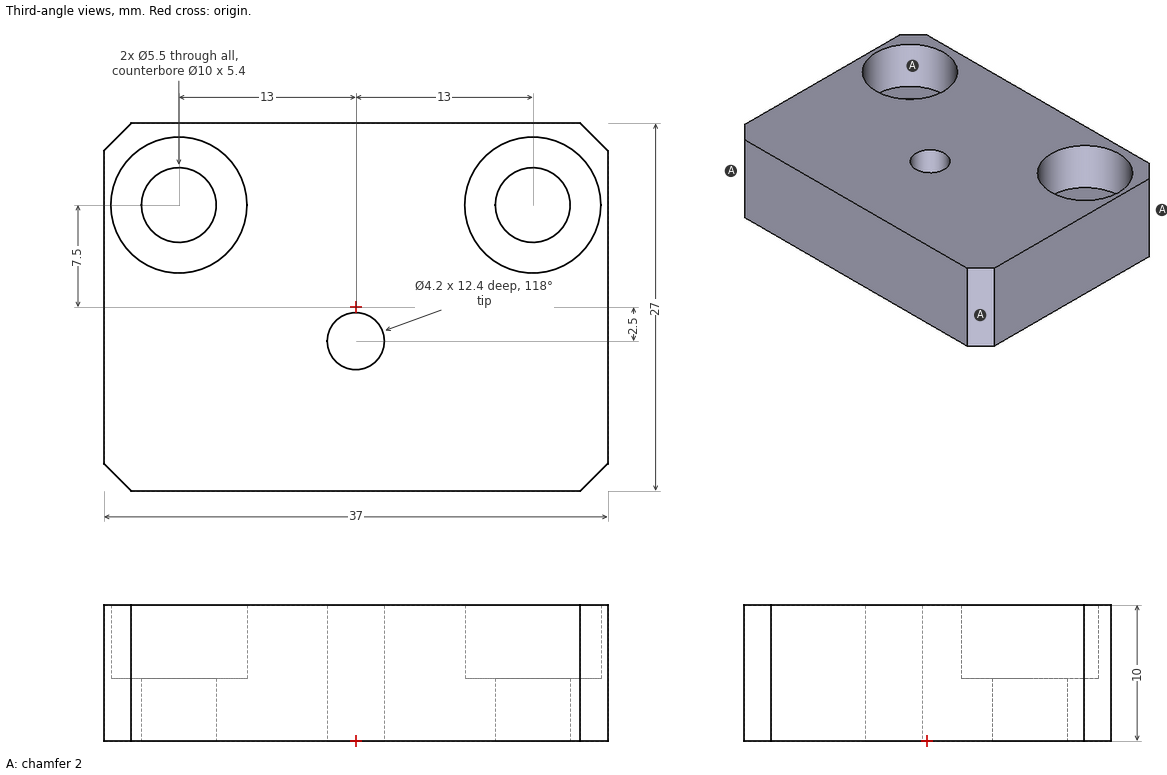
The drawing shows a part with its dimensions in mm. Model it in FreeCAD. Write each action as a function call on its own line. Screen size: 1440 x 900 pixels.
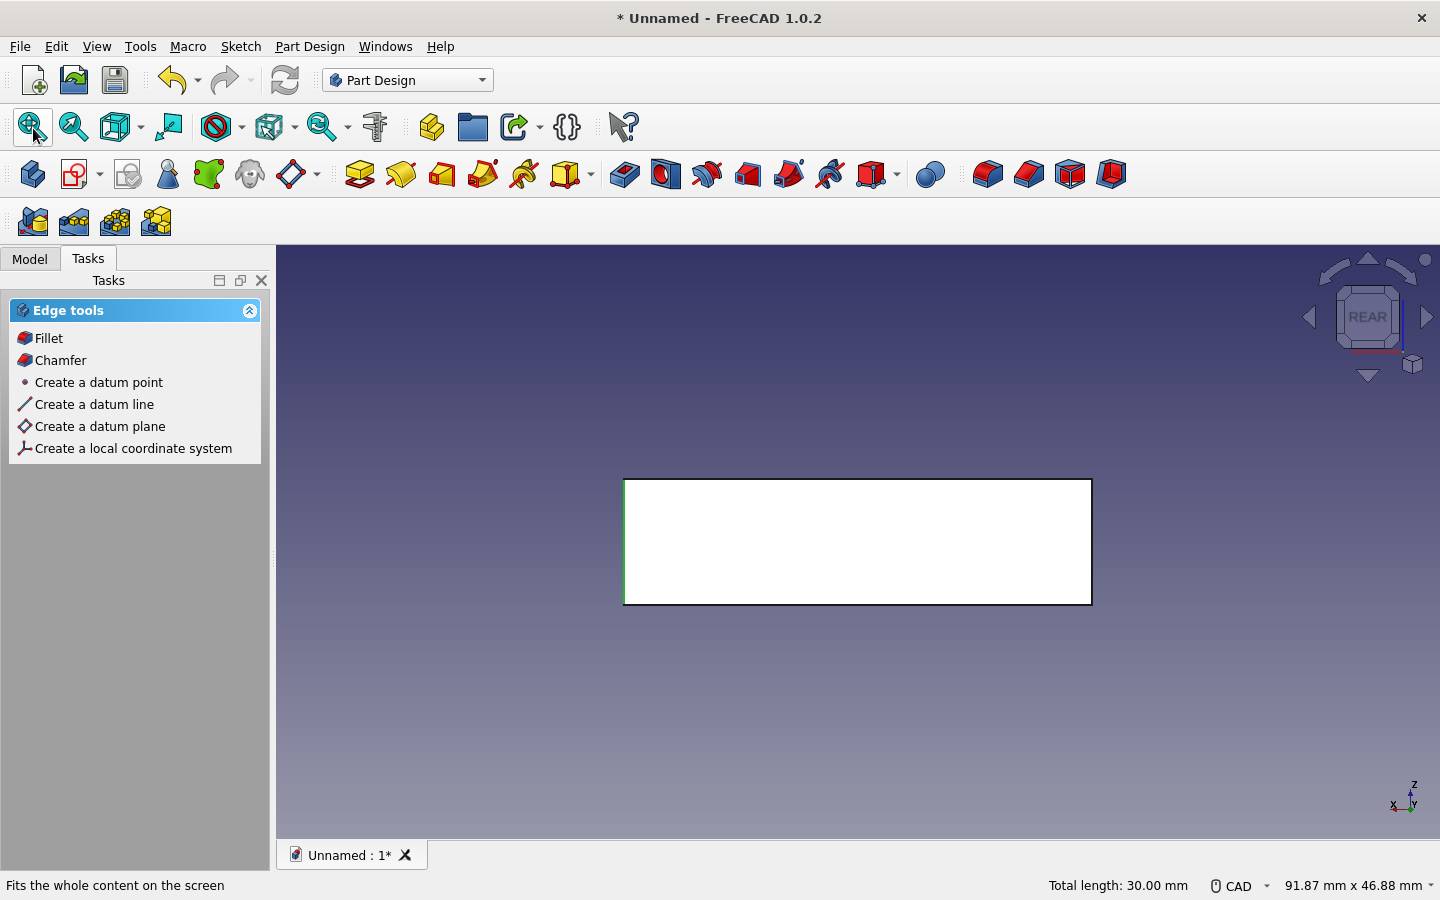
click(1092, 541, ctrl)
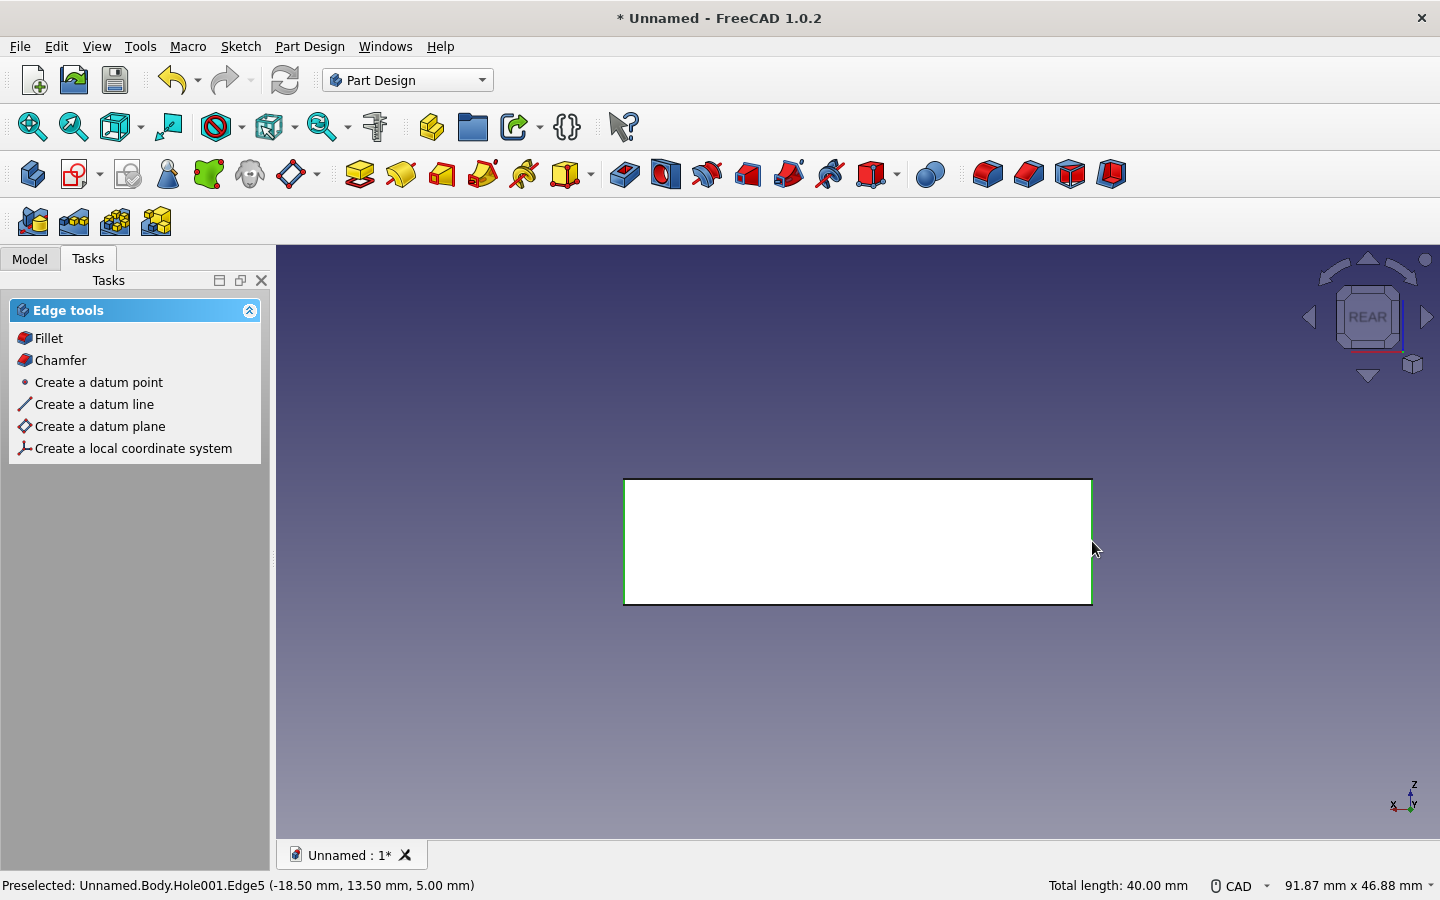
click(1029, 174)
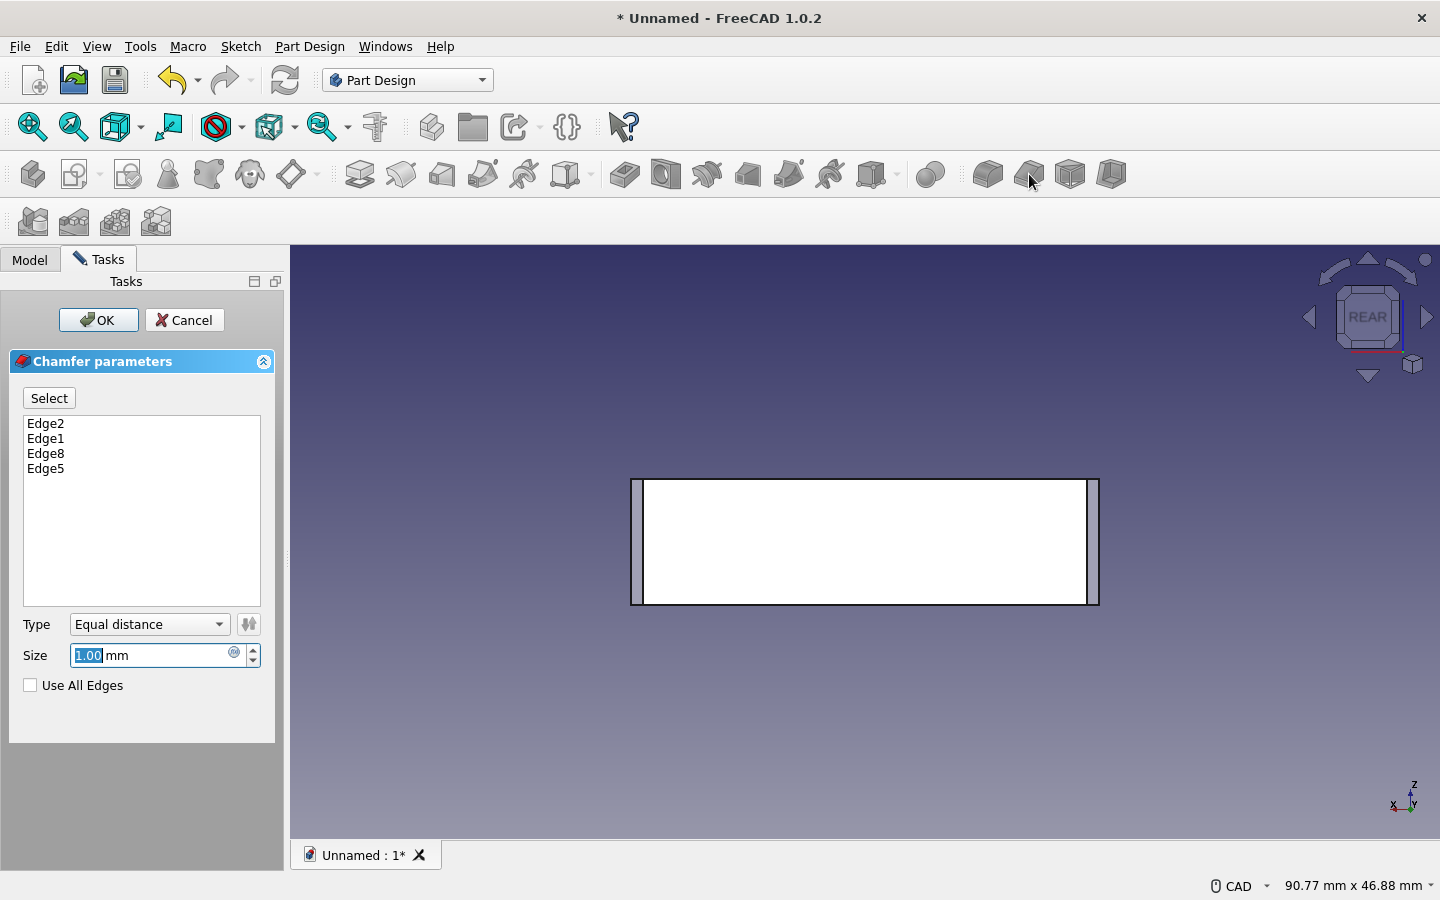
text(2)
key(Tab)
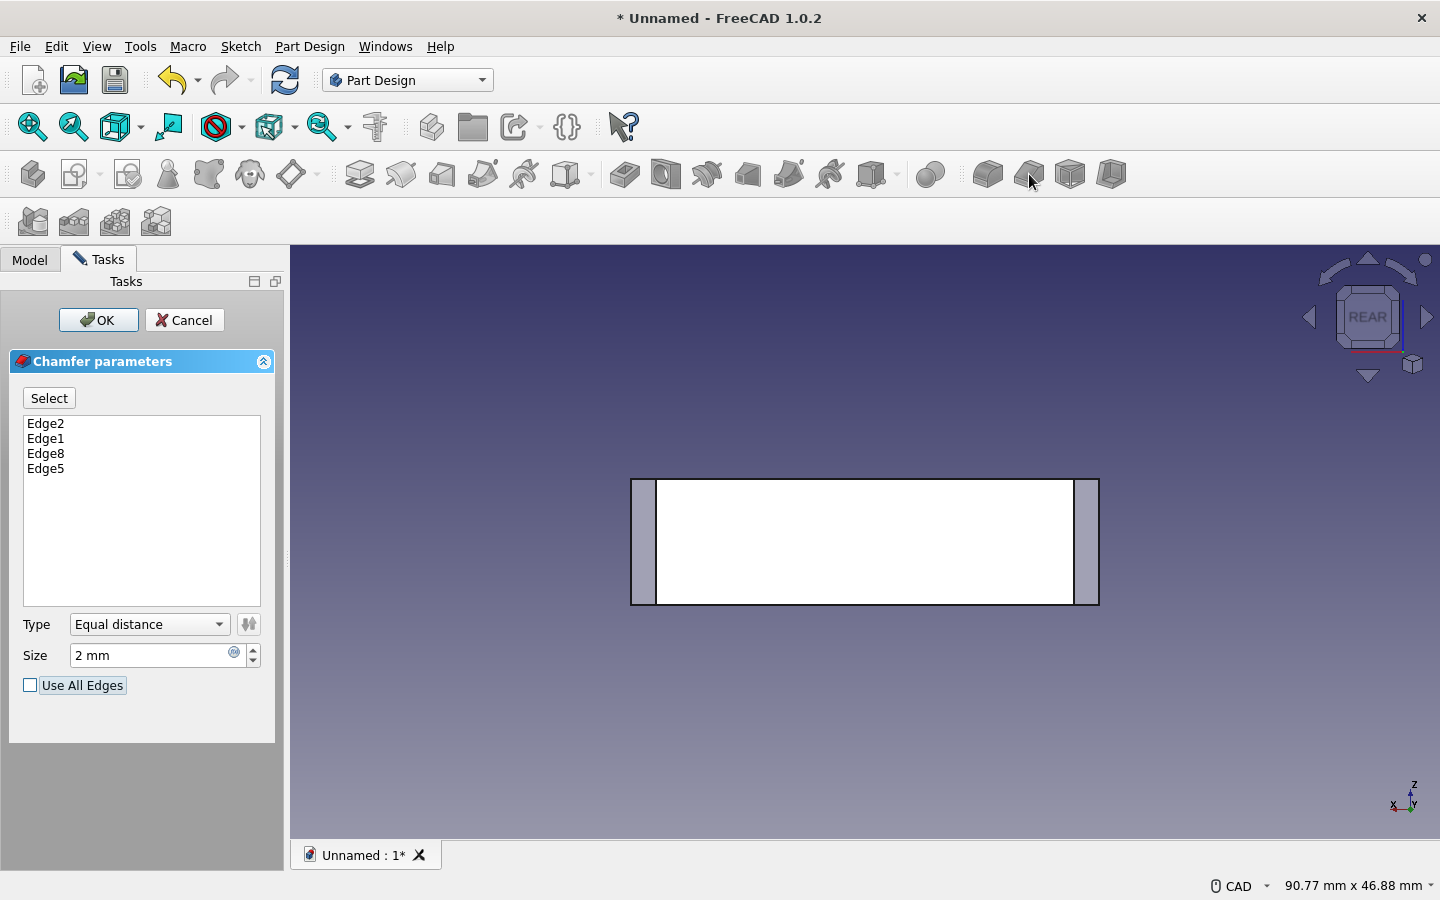
click(99, 320)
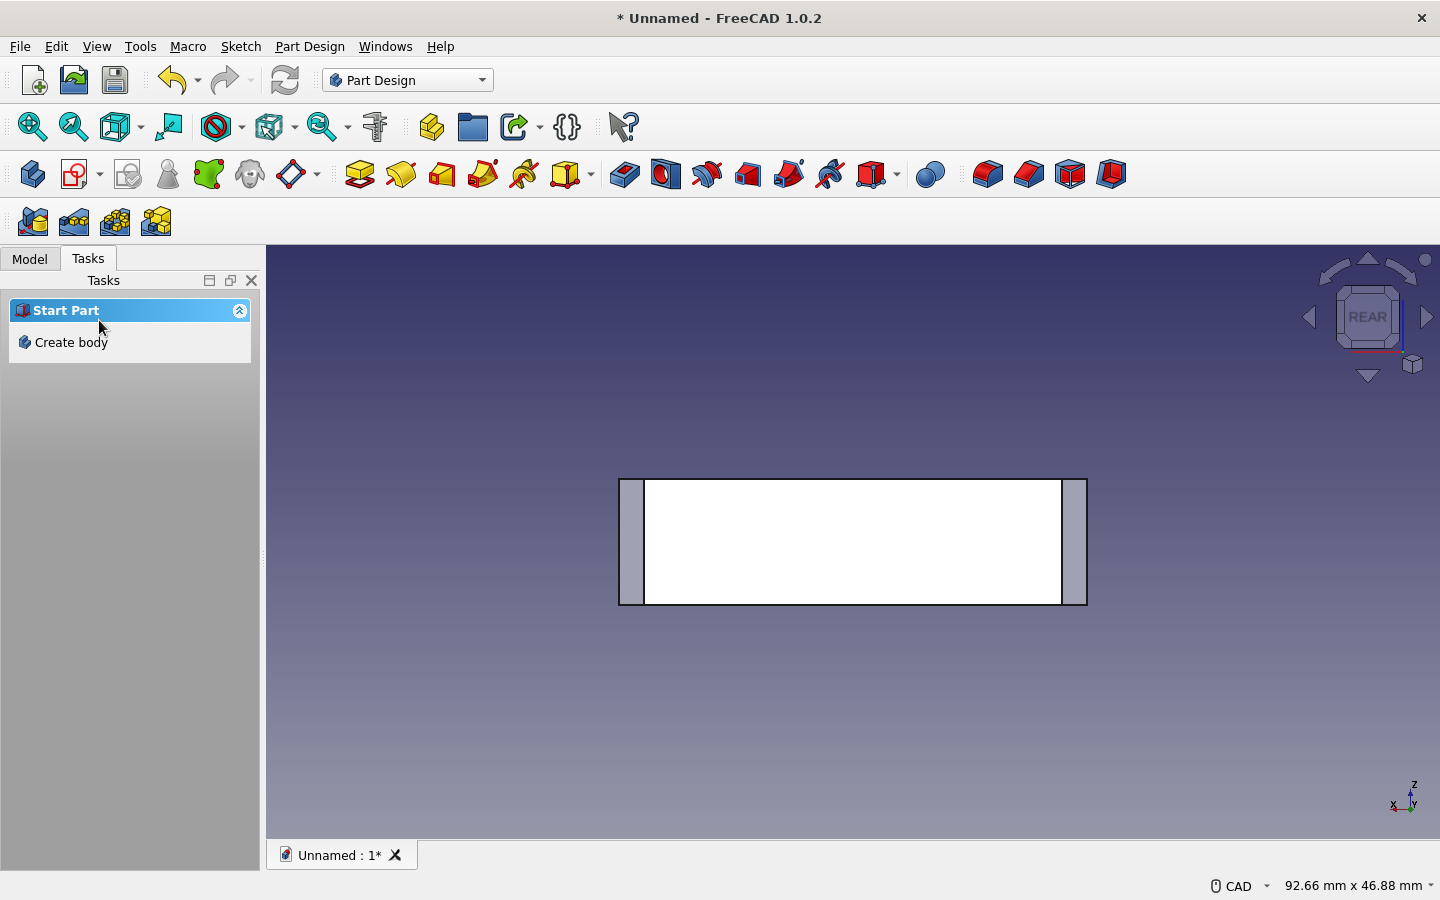
key(0)